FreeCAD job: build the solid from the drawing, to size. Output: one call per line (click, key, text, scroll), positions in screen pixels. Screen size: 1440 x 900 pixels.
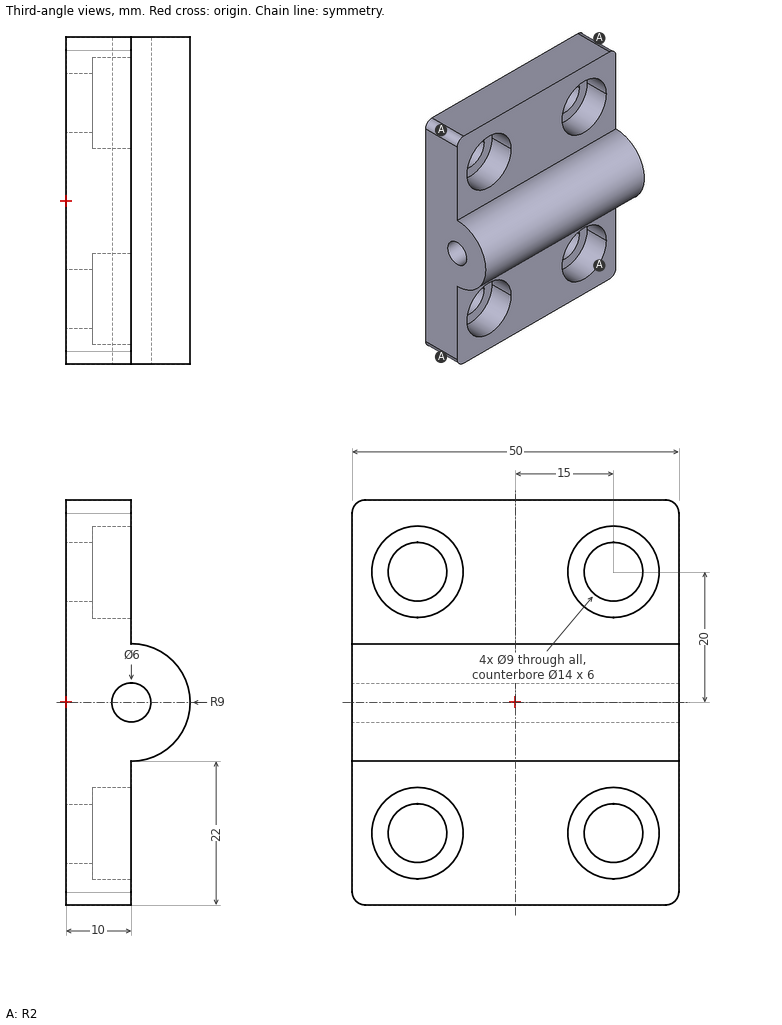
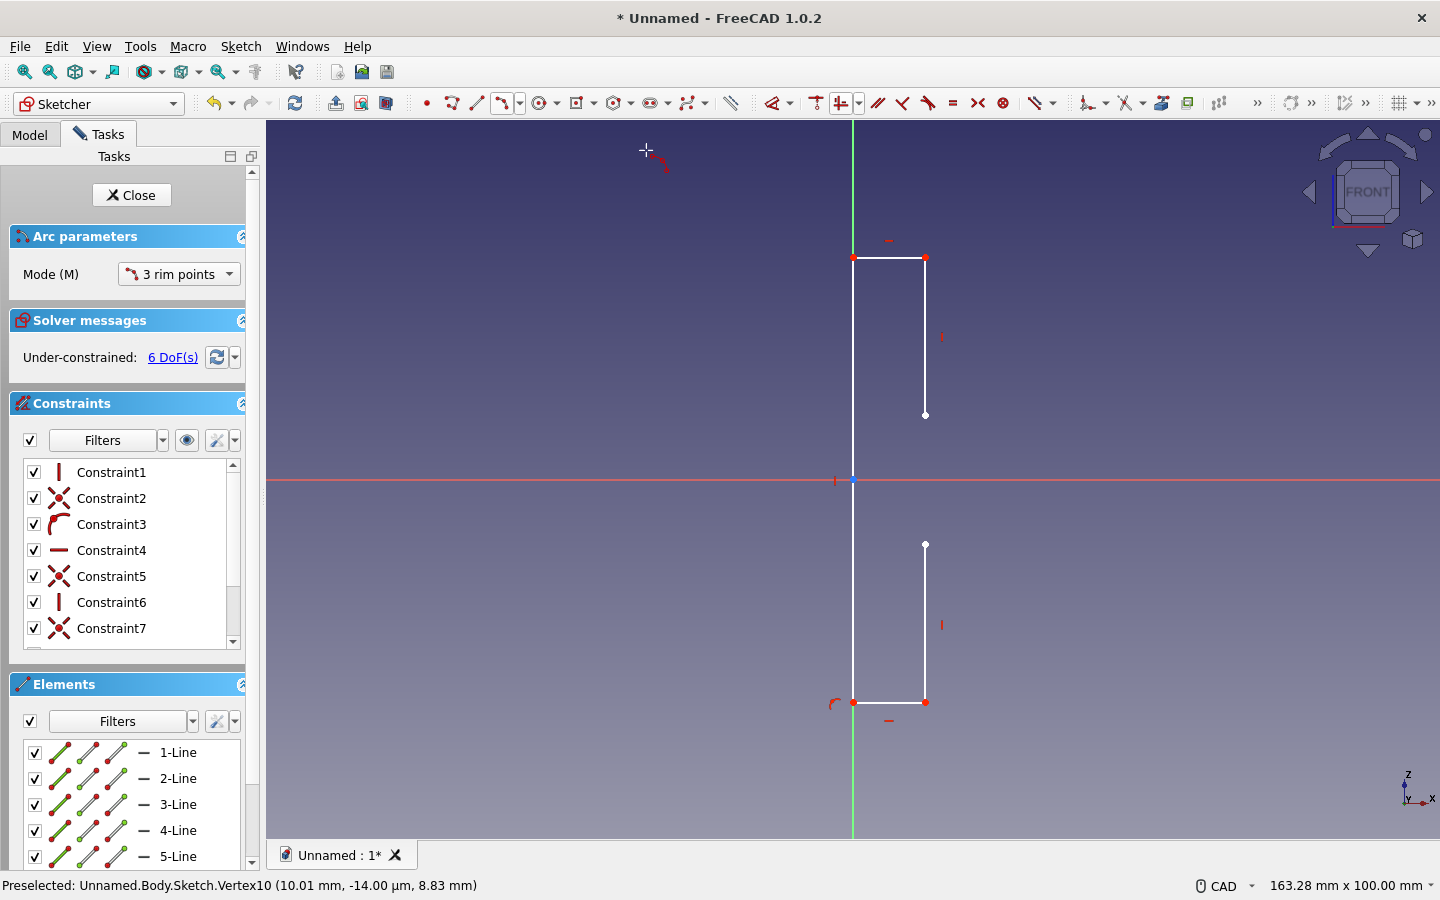
click(925, 416)
click(925, 545)
click(986, 499)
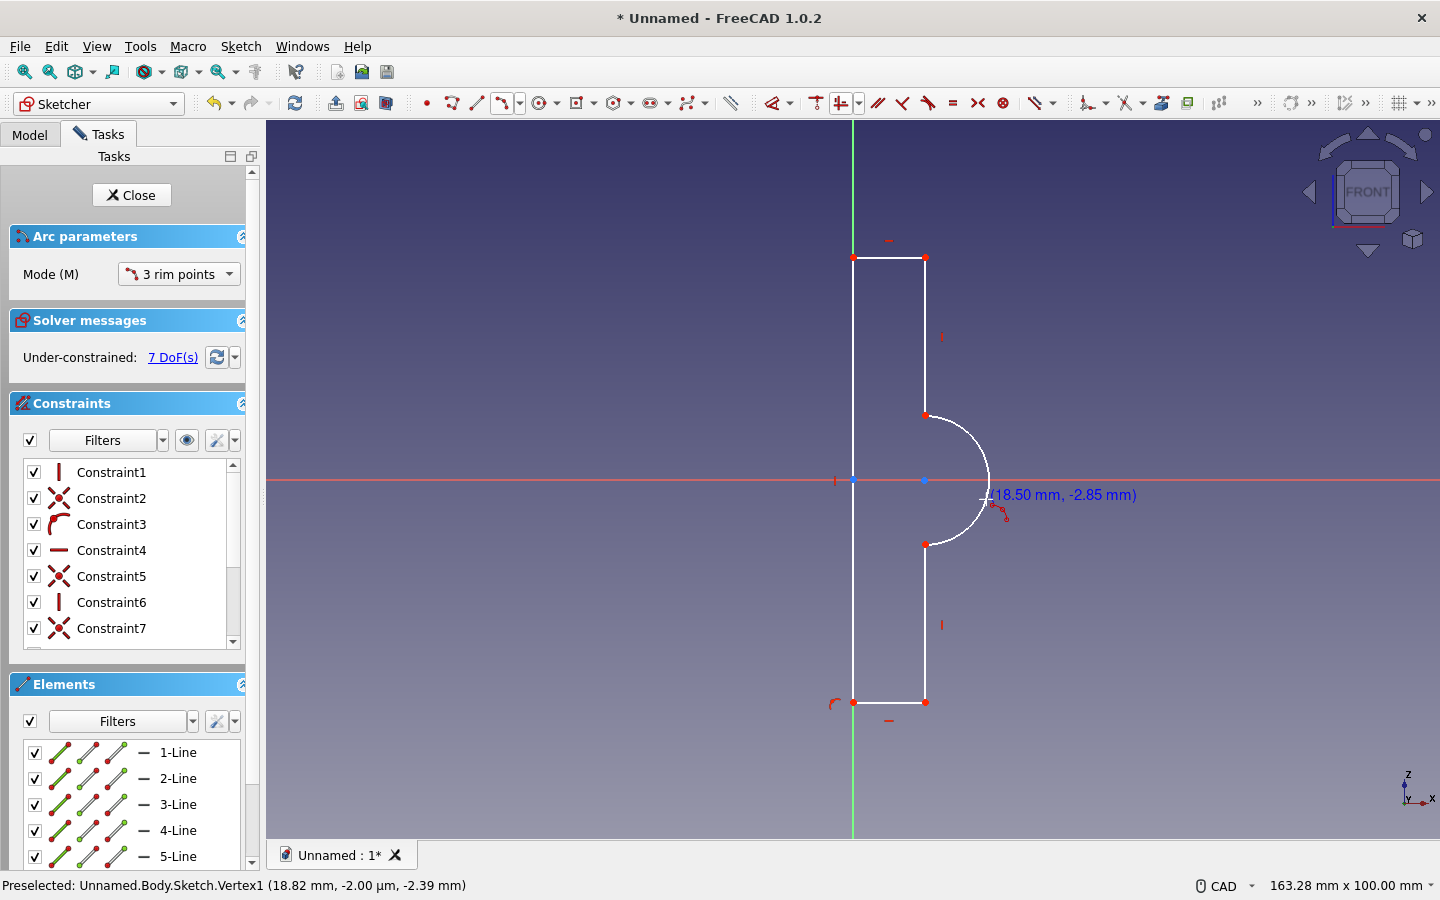
click(538, 104)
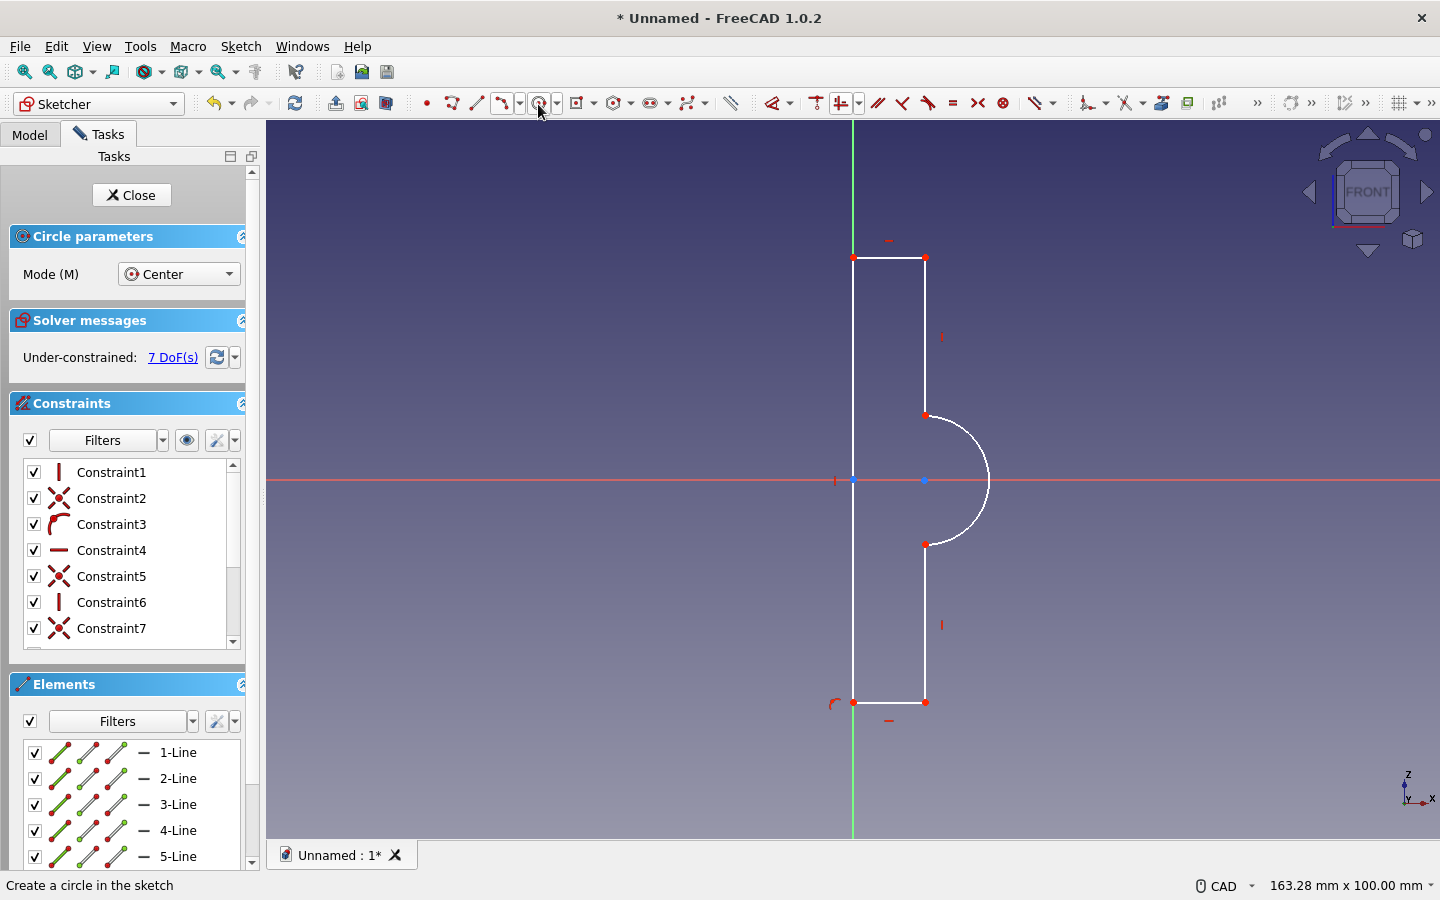
click(925, 480)
move(940, 464)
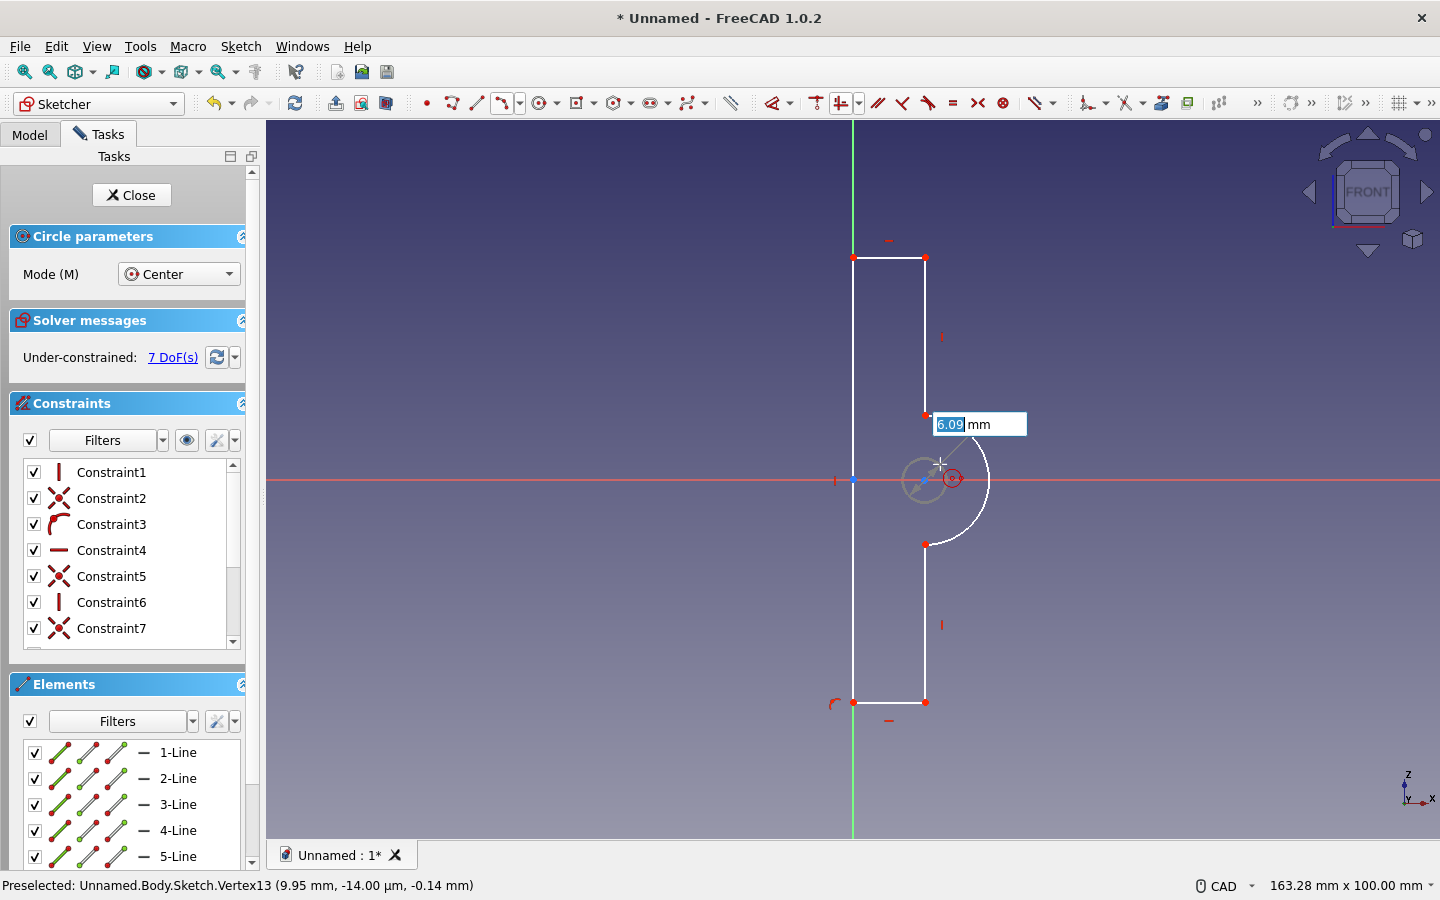
text(6)
key(Return)
key(Escape)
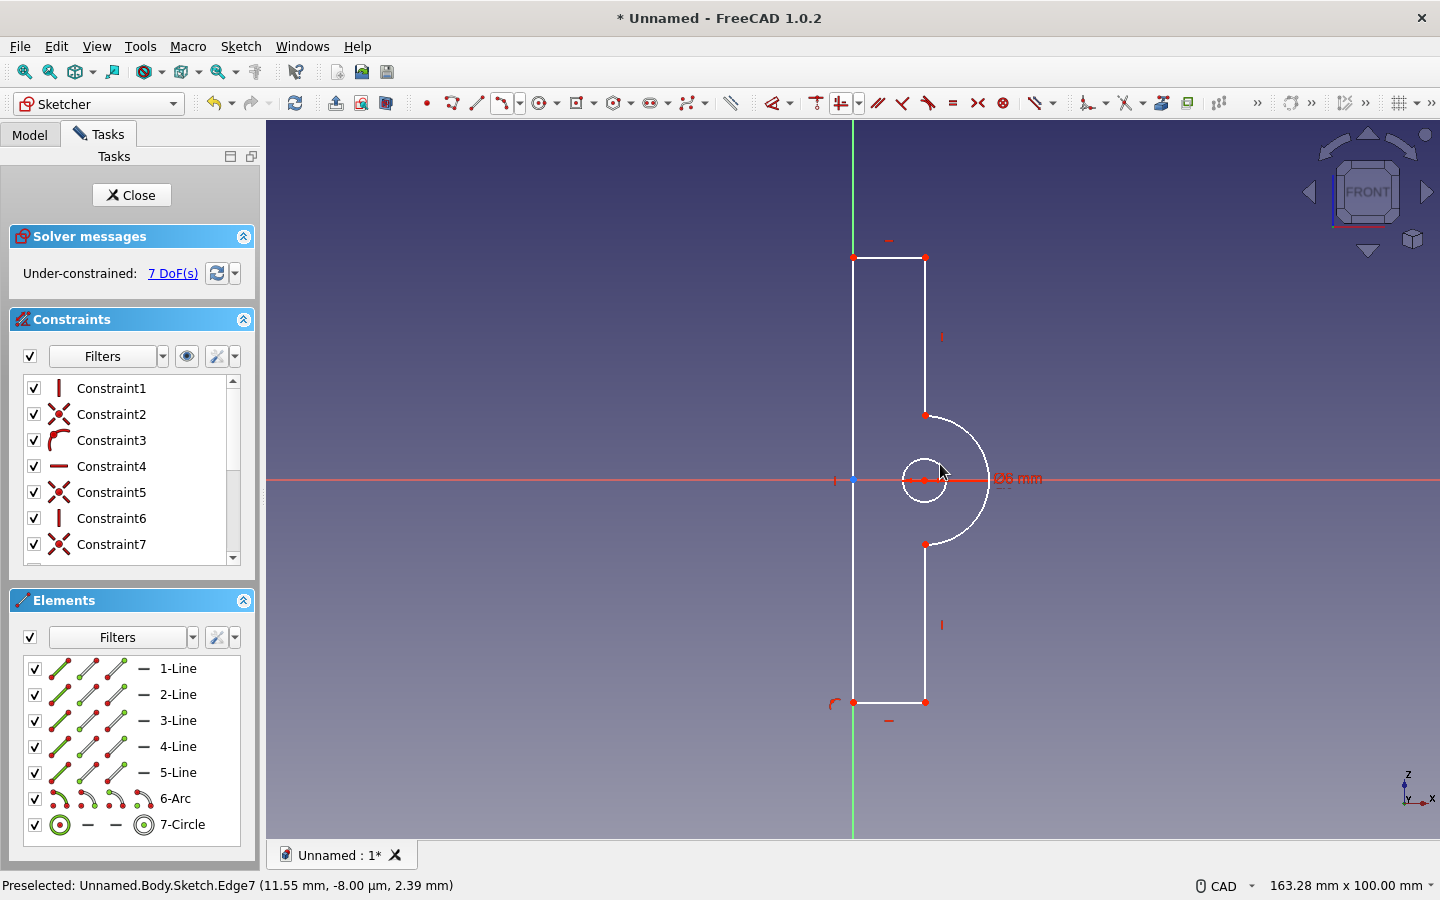
click(925, 481)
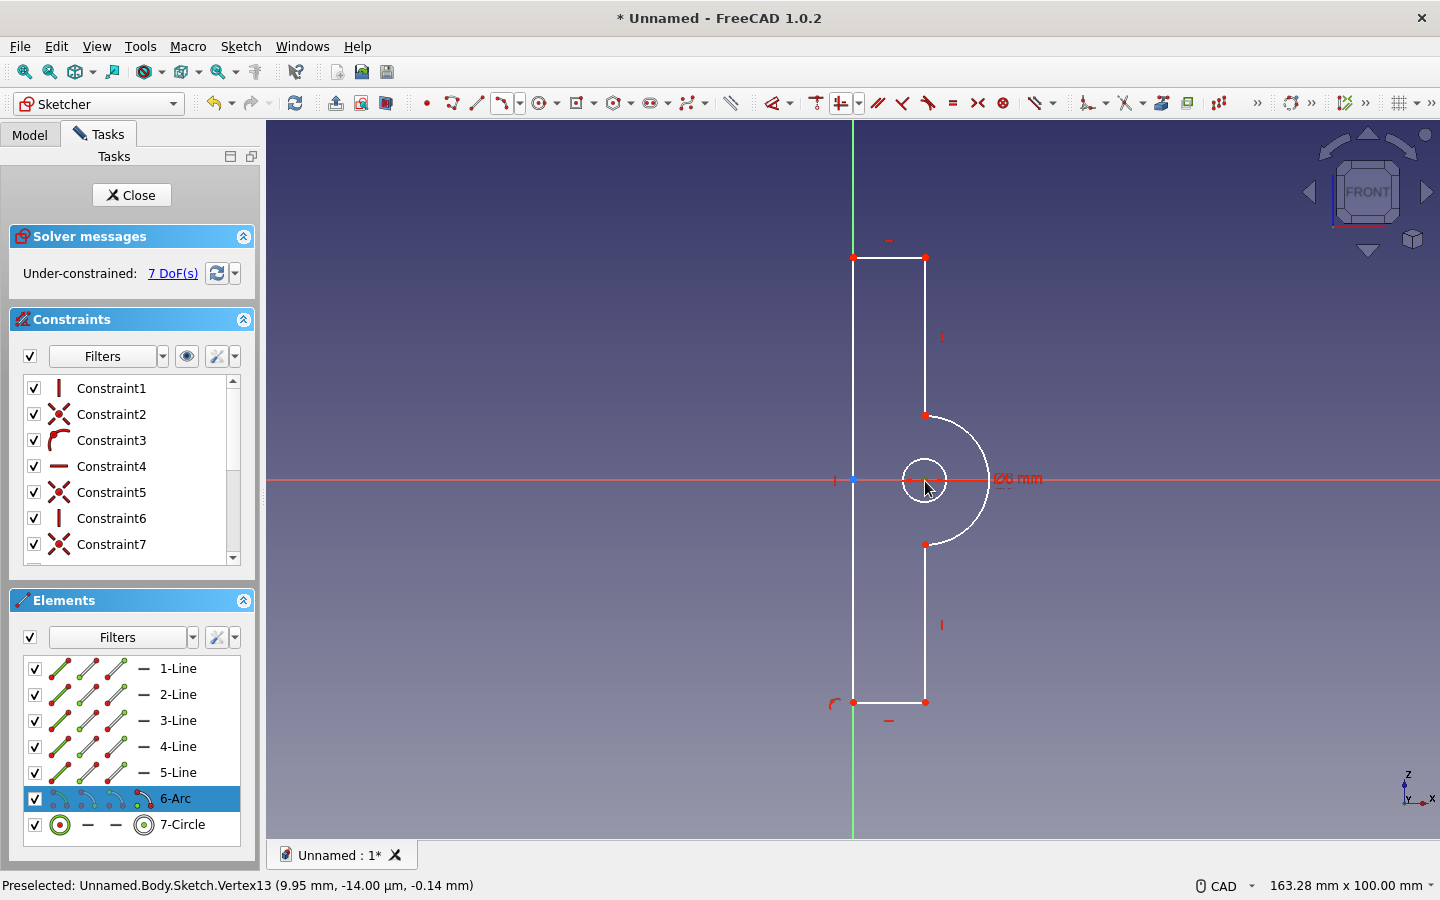
click(364, 480)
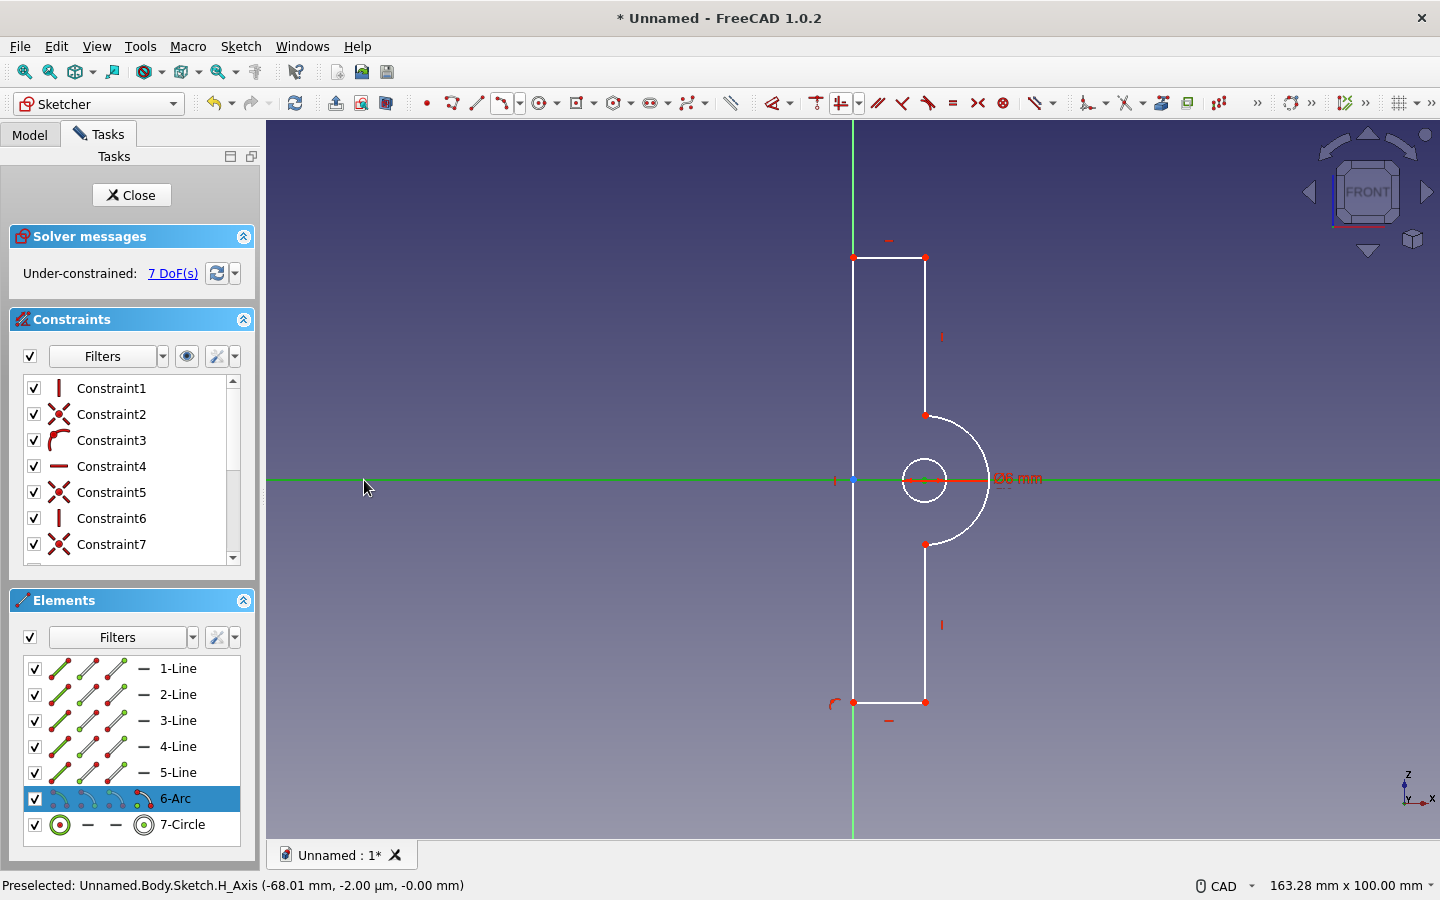
click(816, 104)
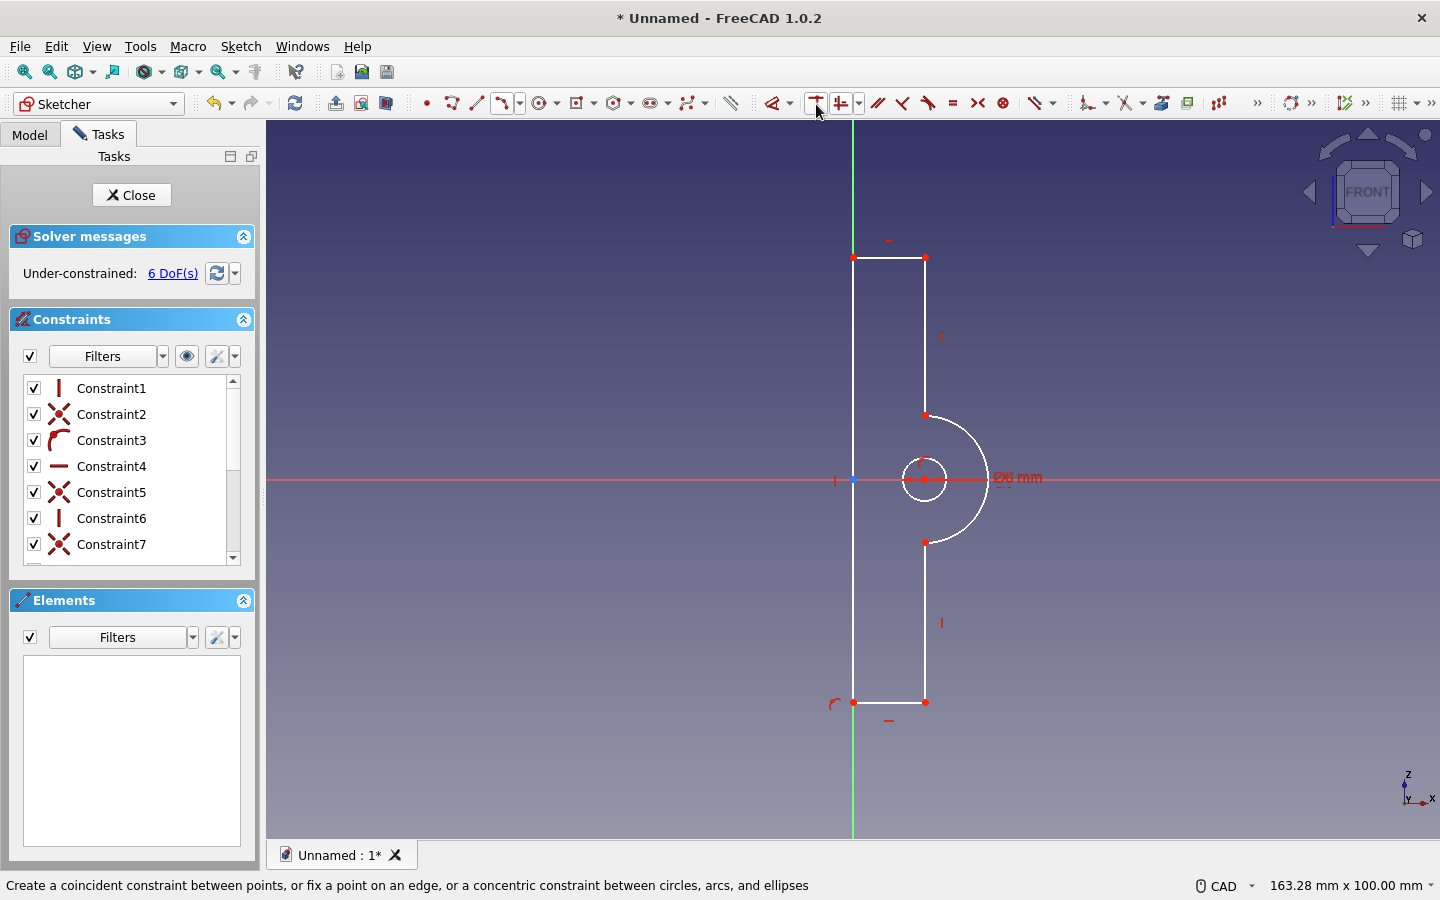
click(925, 703)